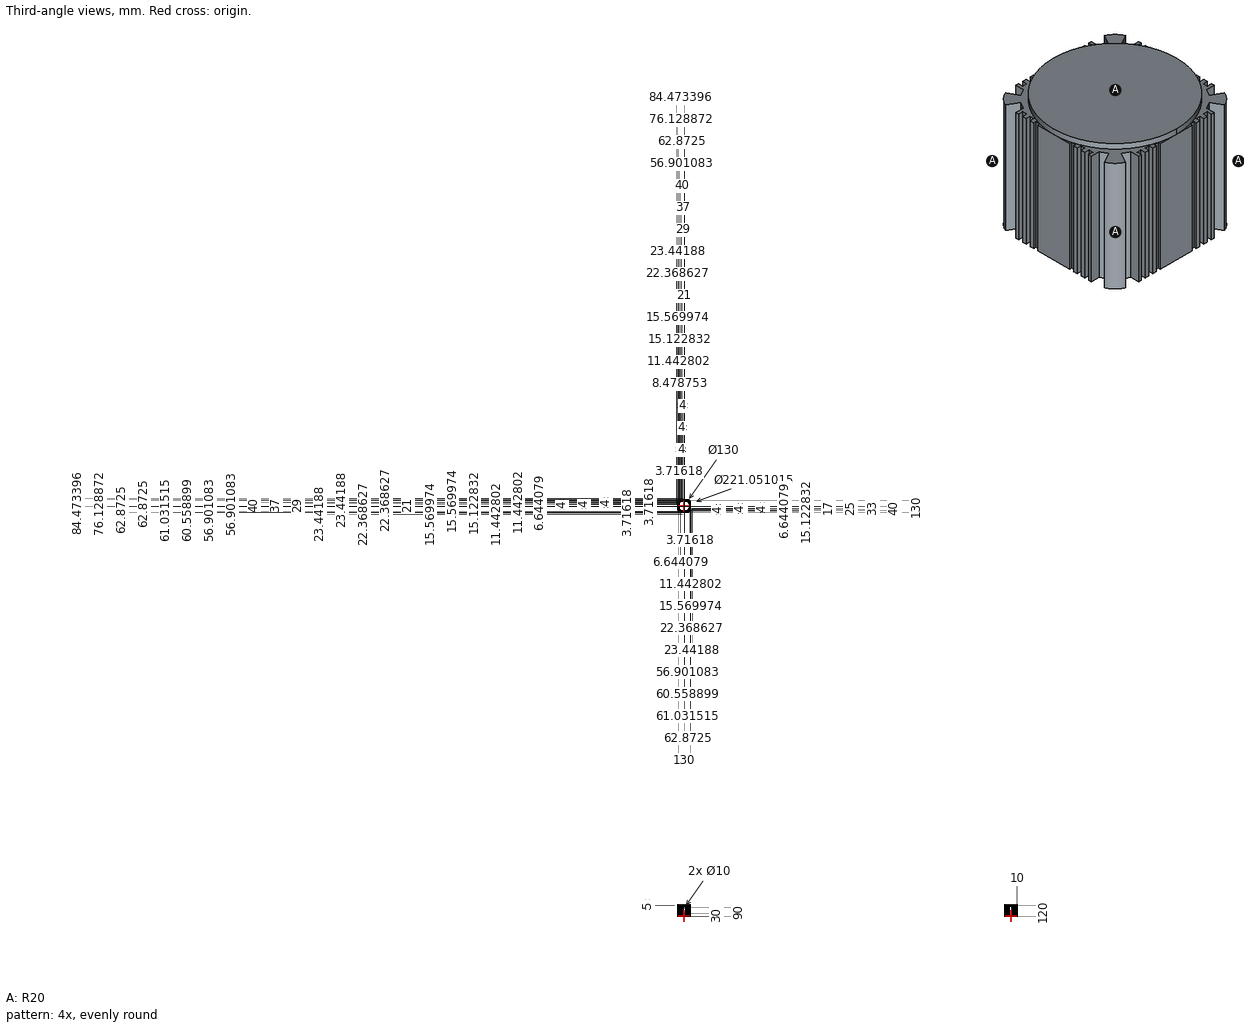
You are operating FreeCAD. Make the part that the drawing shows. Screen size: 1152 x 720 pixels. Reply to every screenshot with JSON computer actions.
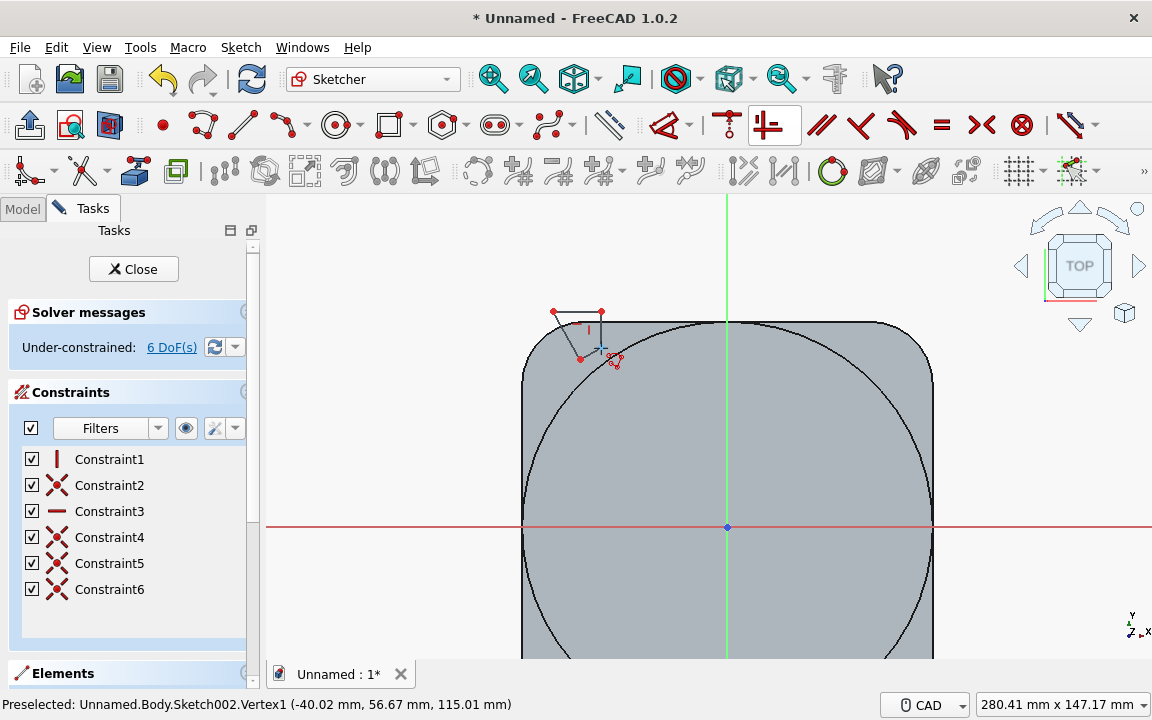
{"action": "left_click", "coordinate": [390, 126]}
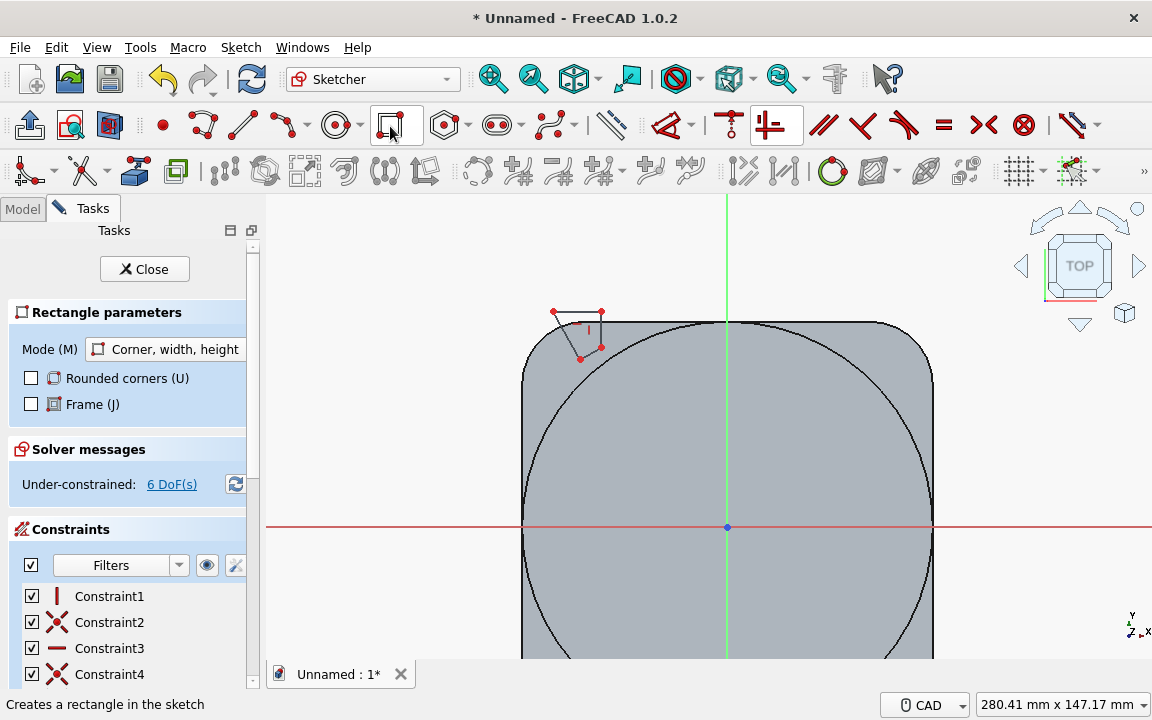
{"action": "scroll", "coordinate": [611, 287], "scroll_direction": "up", "scroll_amount": 2}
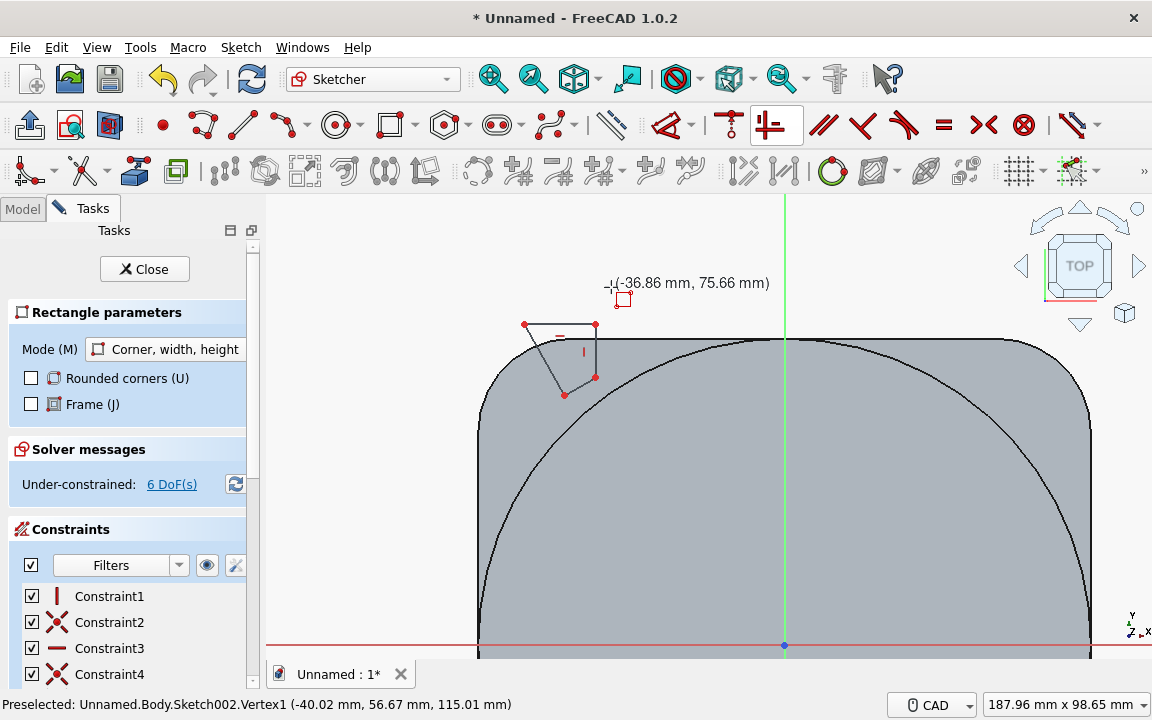
{"action": "left_click", "coordinate": [610, 286]}
{"action": "mouse_move", "coordinate": [629, 360]}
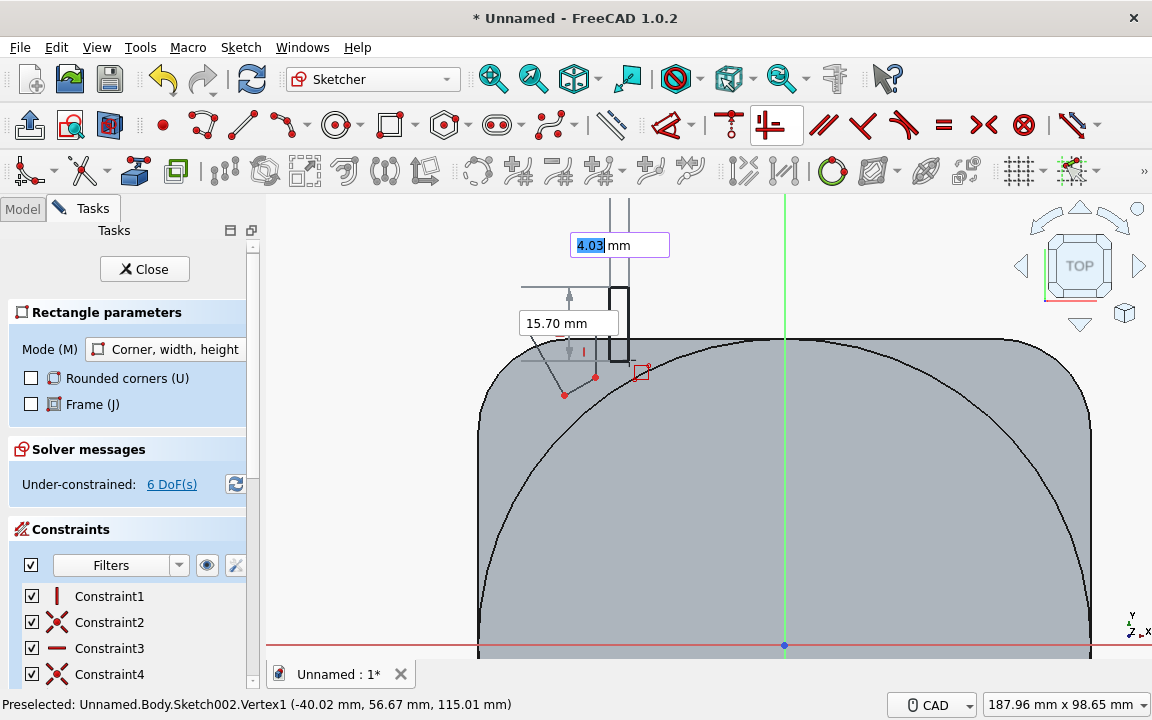
{"action": "type", "text": "4"}
{"action": "key", "text": "Tab"}
{"action": "type", "text": "15.569974"}
{"action": "key", "text": "Return"}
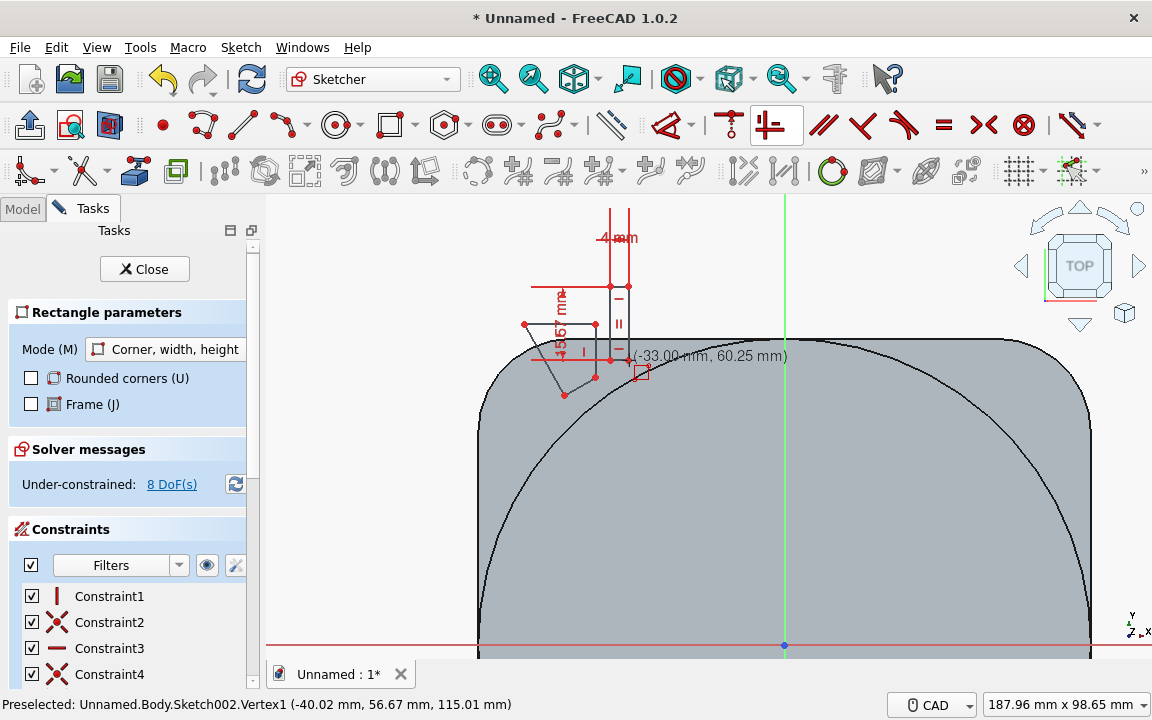
{"action": "left_click", "coordinate": [648, 247]}
{"action": "mouse_move", "coordinate": [667, 357]}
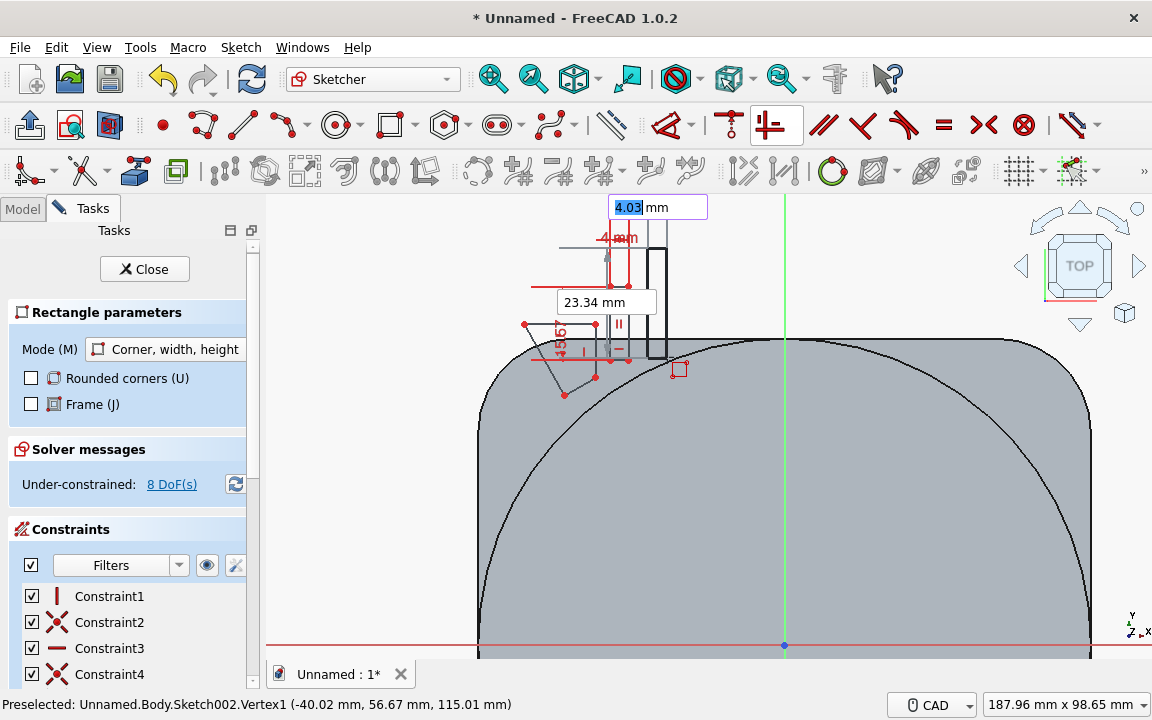
{"action": "type", "text": "4"}
{"action": "key", "text": "Tab"}
{"action": "type", "text": "23.44188"}
{"action": "key", "text": "Return"}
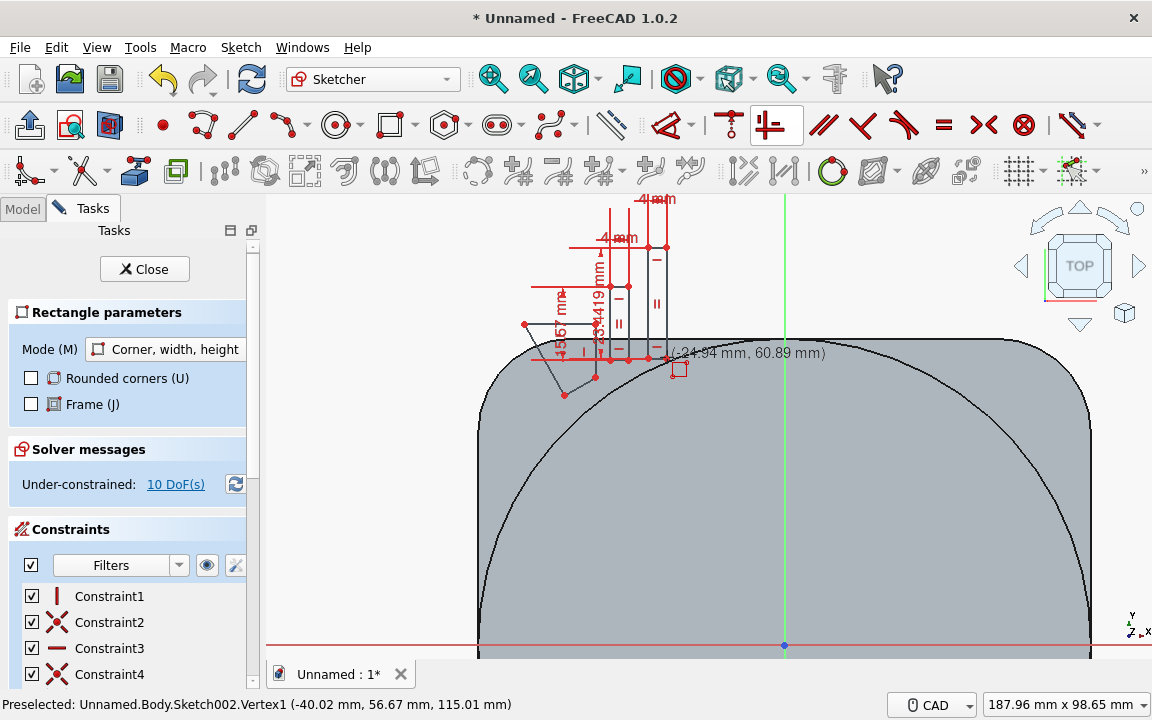
{"action": "left_click", "coordinate": [686, 243]}
{"action": "mouse_move", "coordinate": [704, 349]}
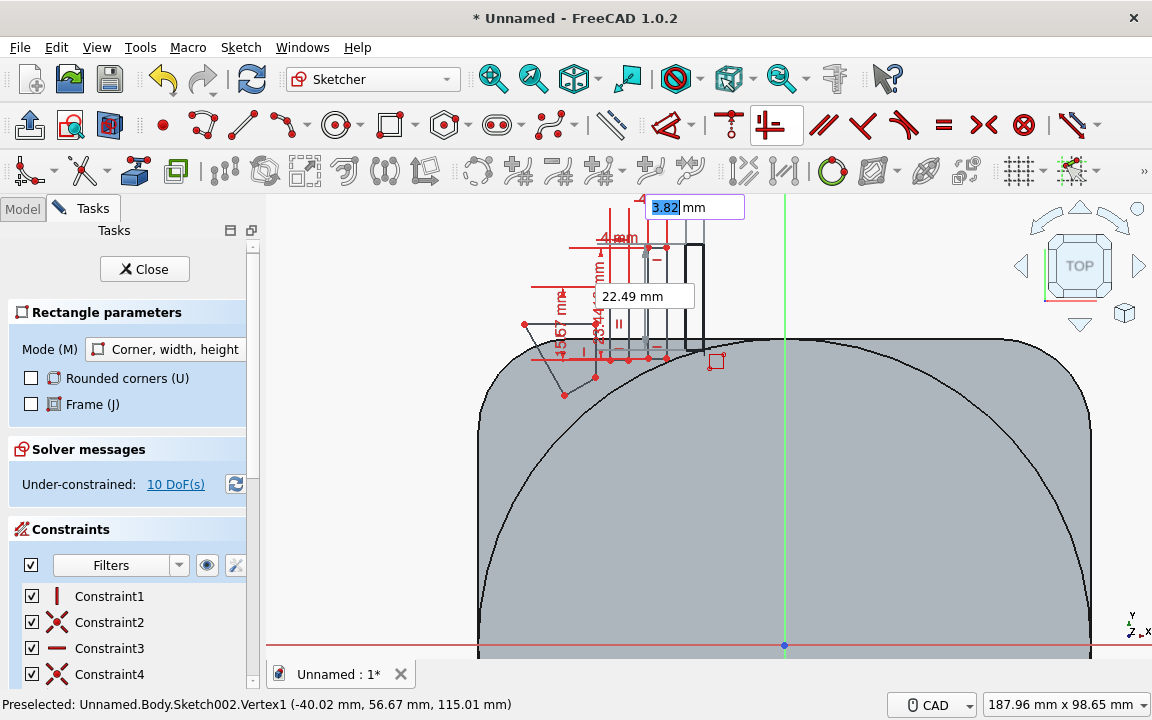
{"action": "type", "text": "4"}
{"action": "key", "text": "Tab"}
{"action": "type", "text": "22.368627"}
{"action": "key", "text": "Return"}
{"action": "key", "text": "Escape"}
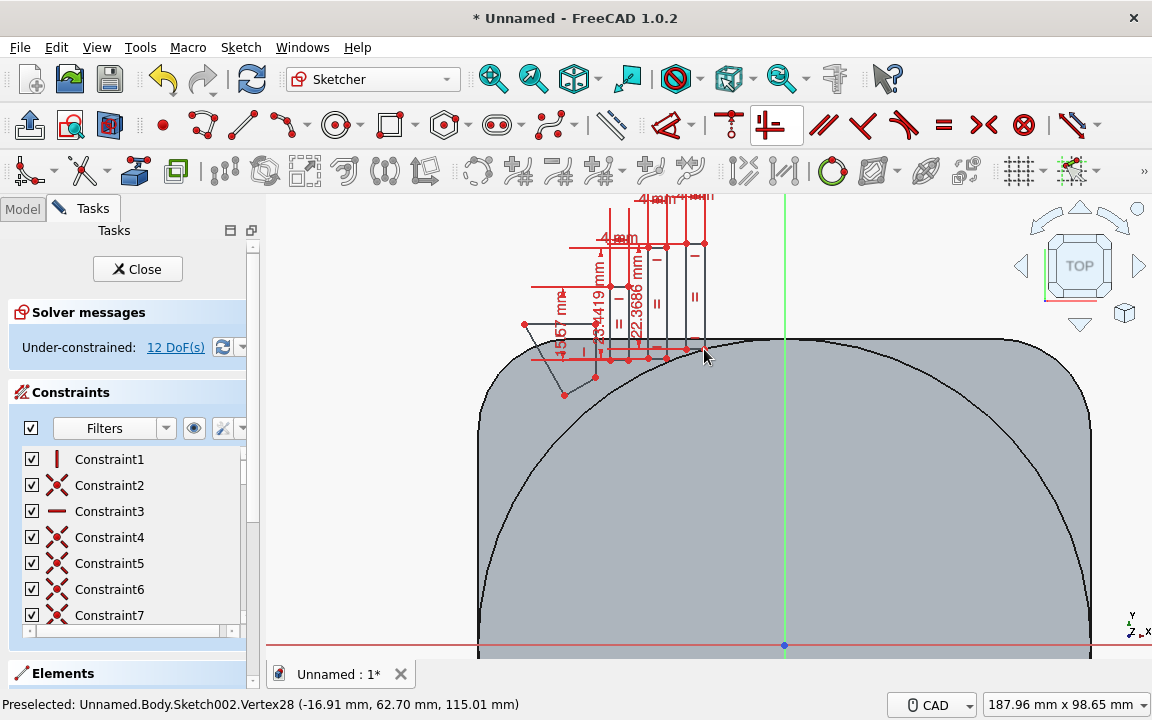
{"action": "left_click", "coordinate": [666, 126]}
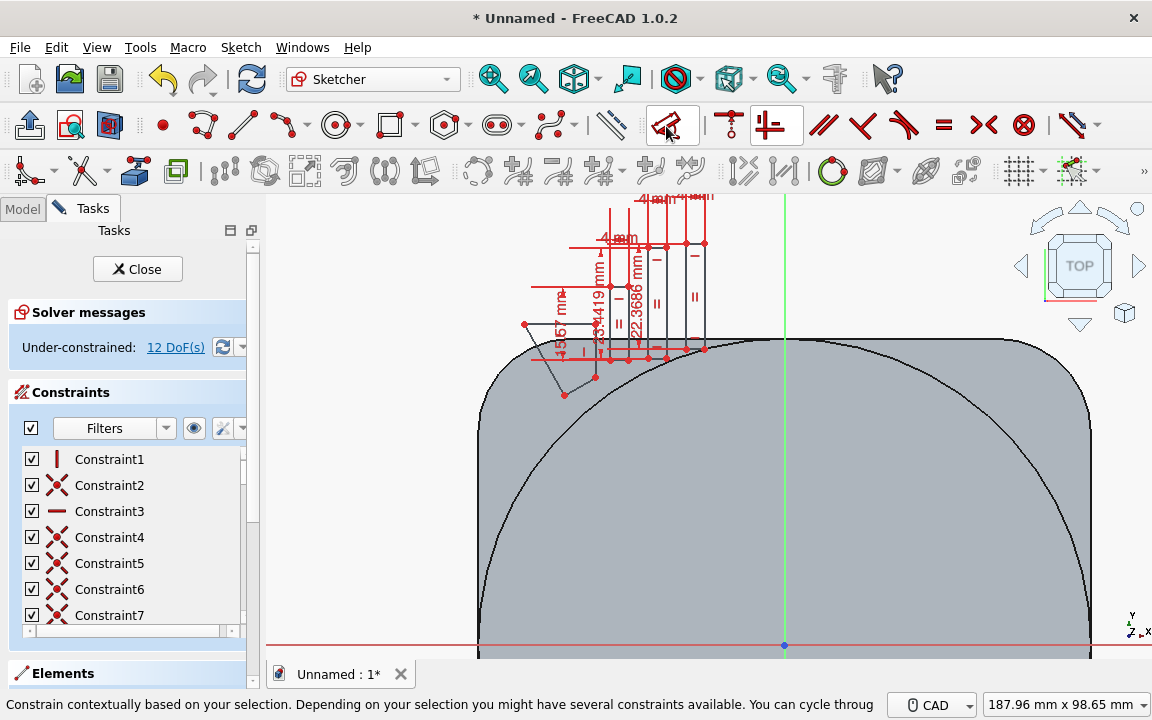
{"action": "left_click", "coordinate": [596, 378]}
{"action": "left_click", "coordinate": [734, 344]}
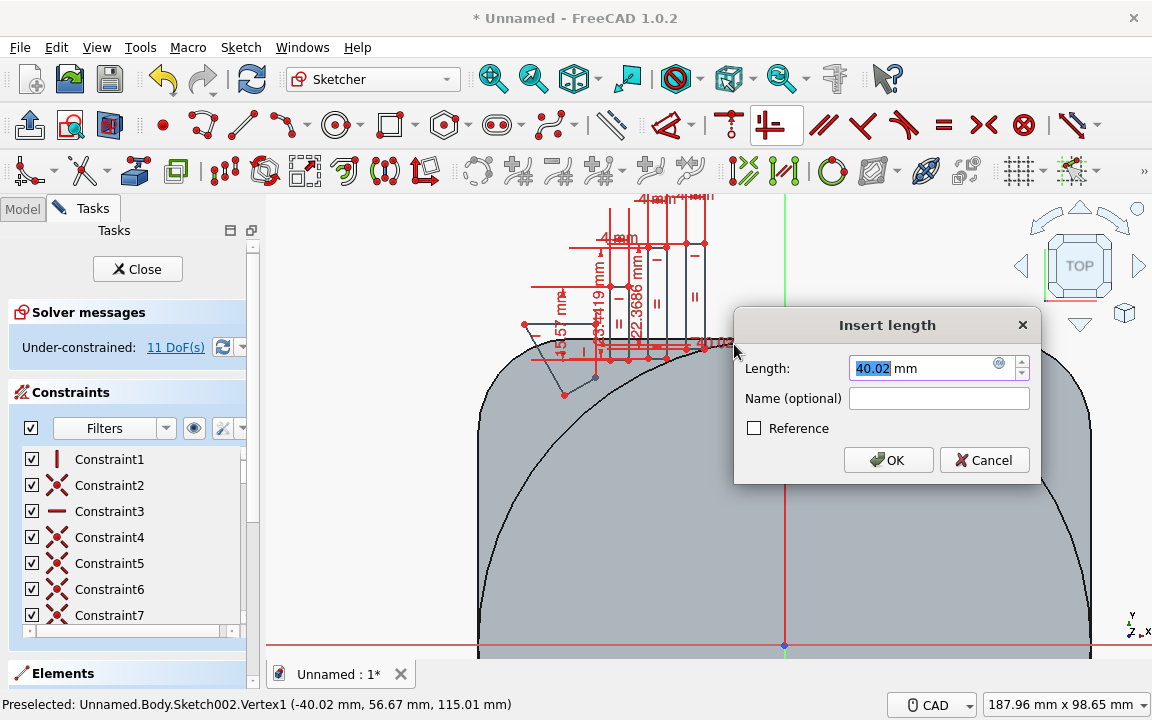
{"action": "type", "text": "40"}
{"action": "key", "text": "Return"}